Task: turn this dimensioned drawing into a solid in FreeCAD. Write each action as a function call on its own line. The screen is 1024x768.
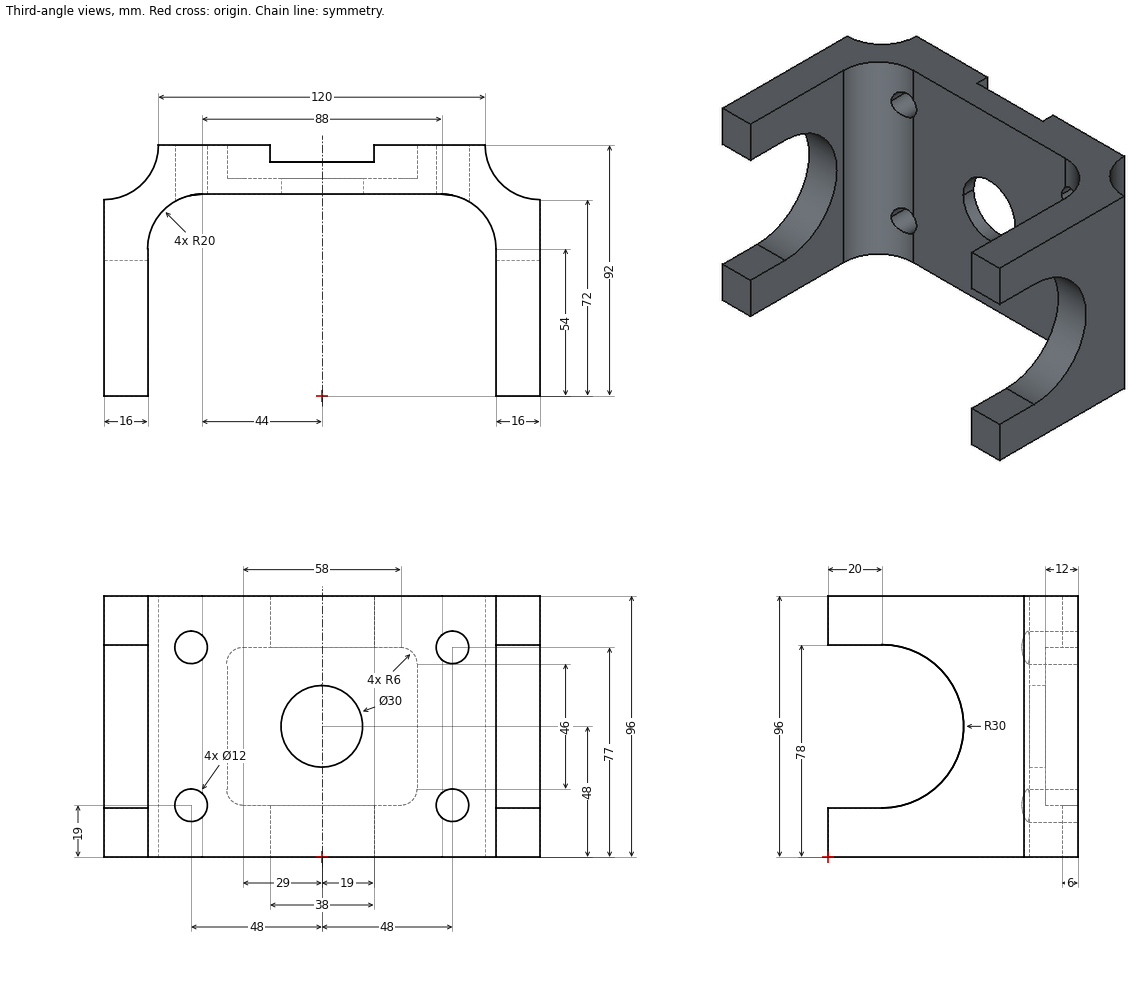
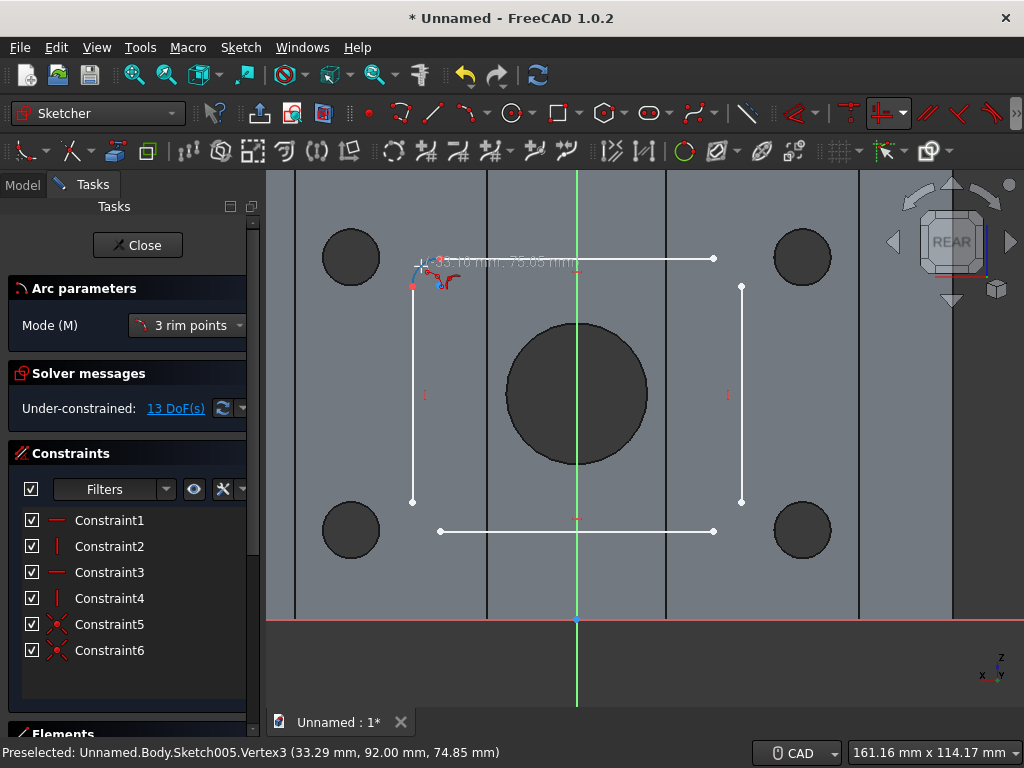
click(413, 503)
click(441, 532)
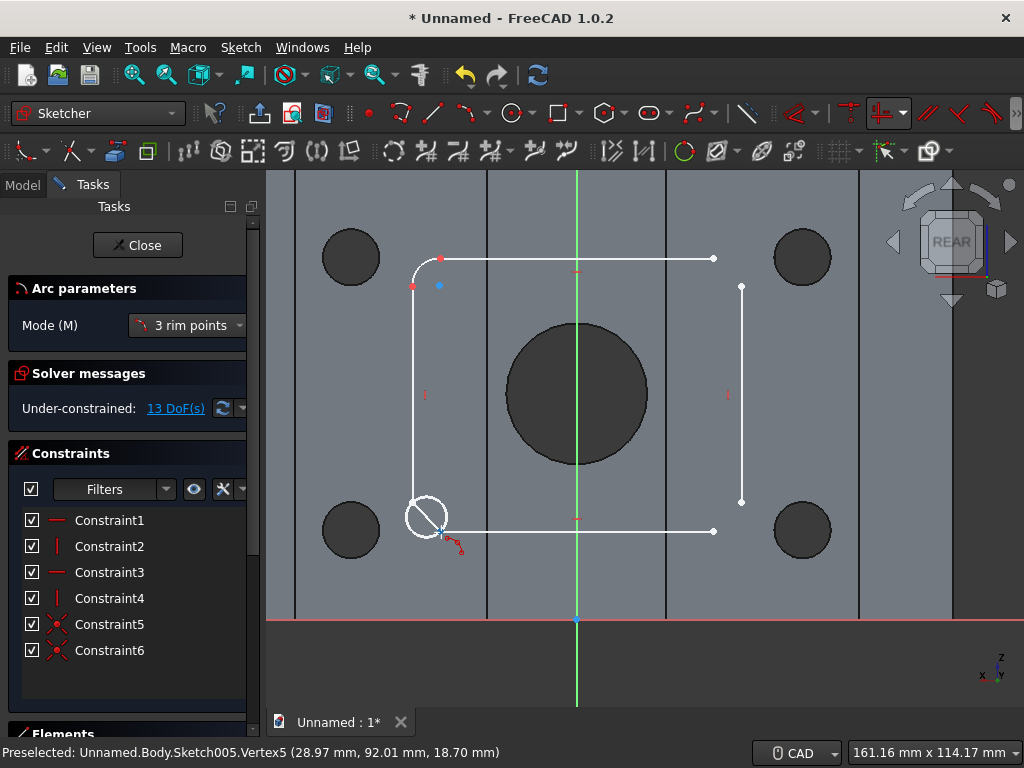
scroll(420, 522, up, 4)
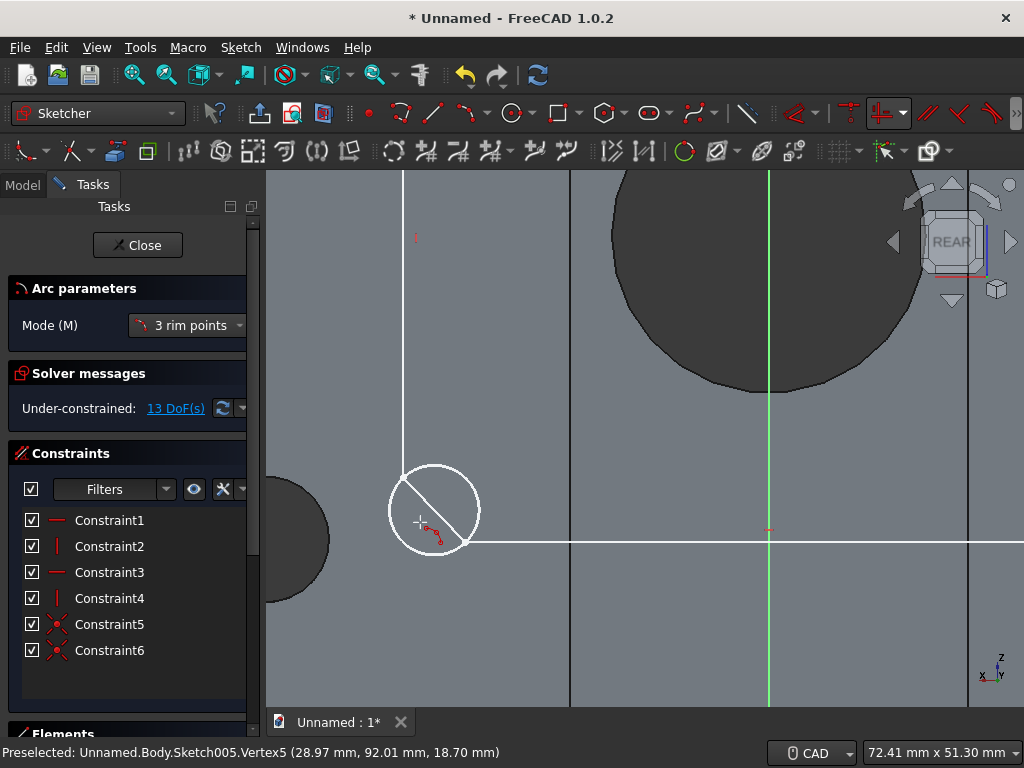
click(421, 521)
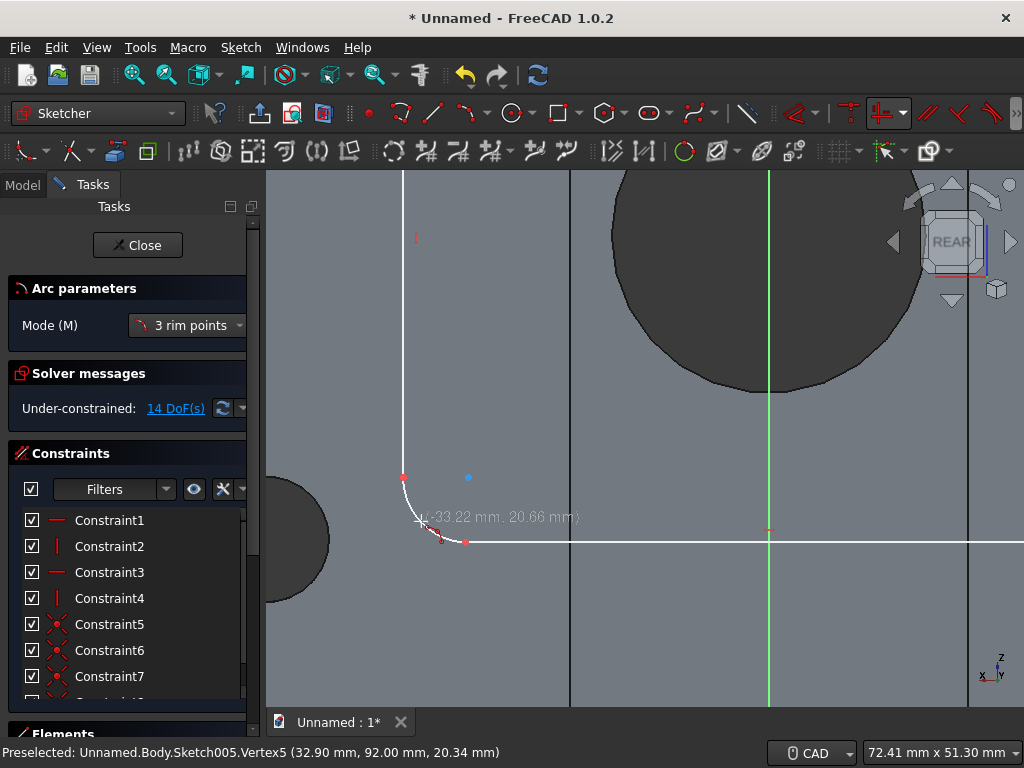
scroll(420, 523, down, 4)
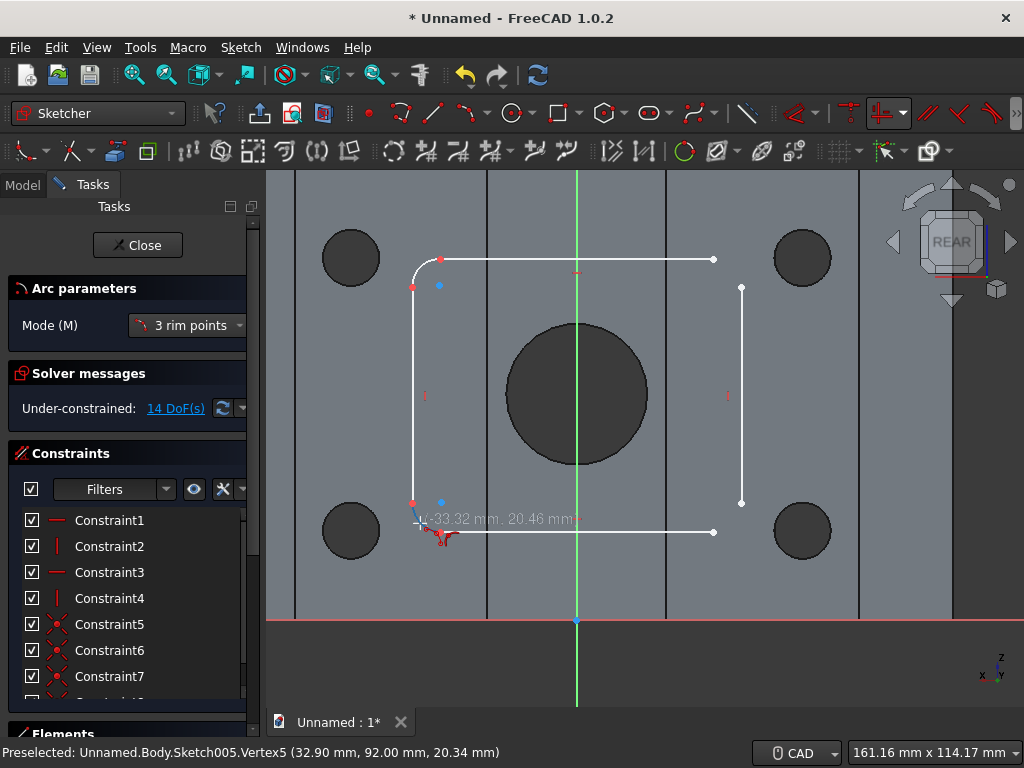
click(714, 532)
click(742, 503)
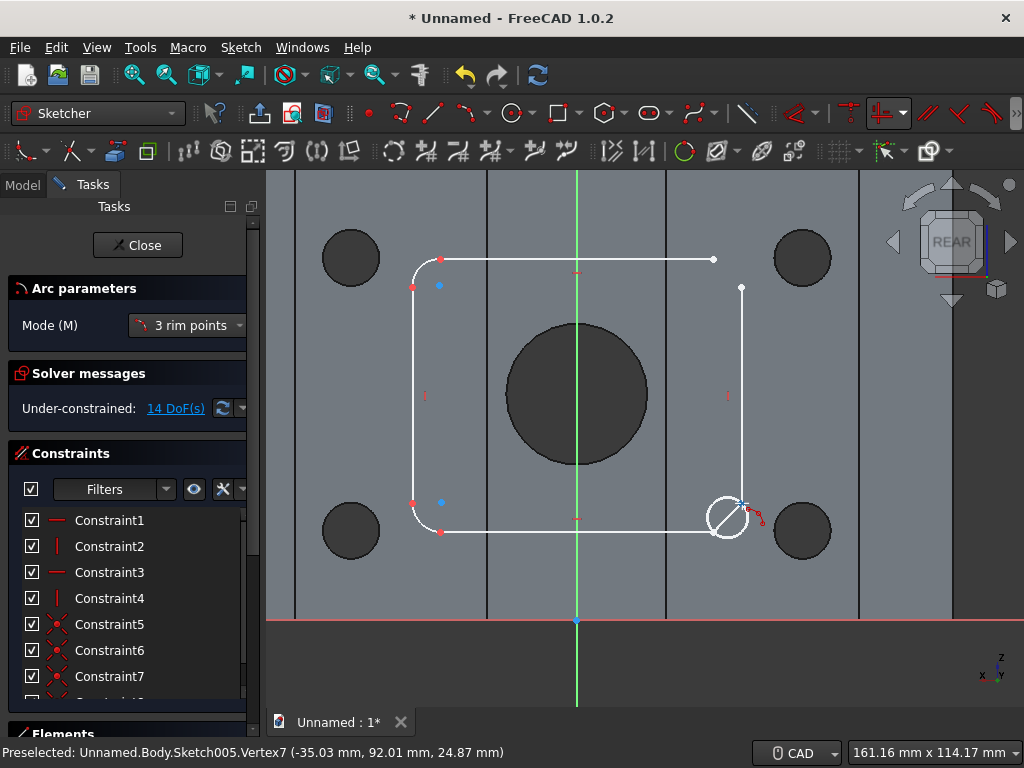
scroll(733, 522, up, 4)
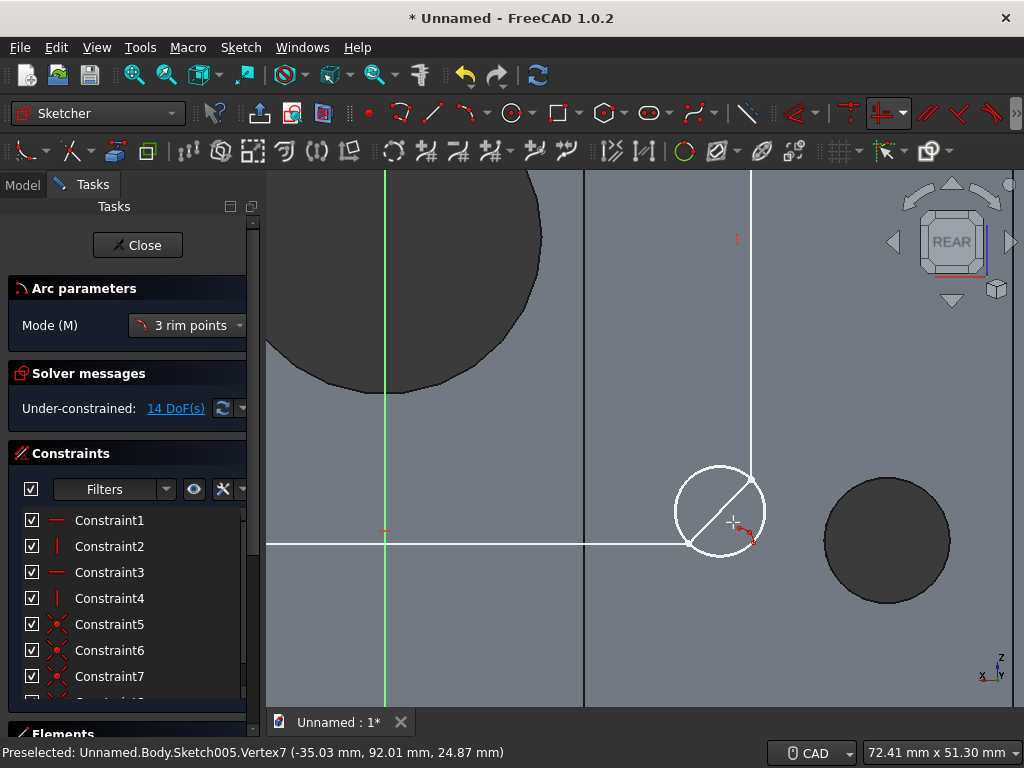
click(733, 522)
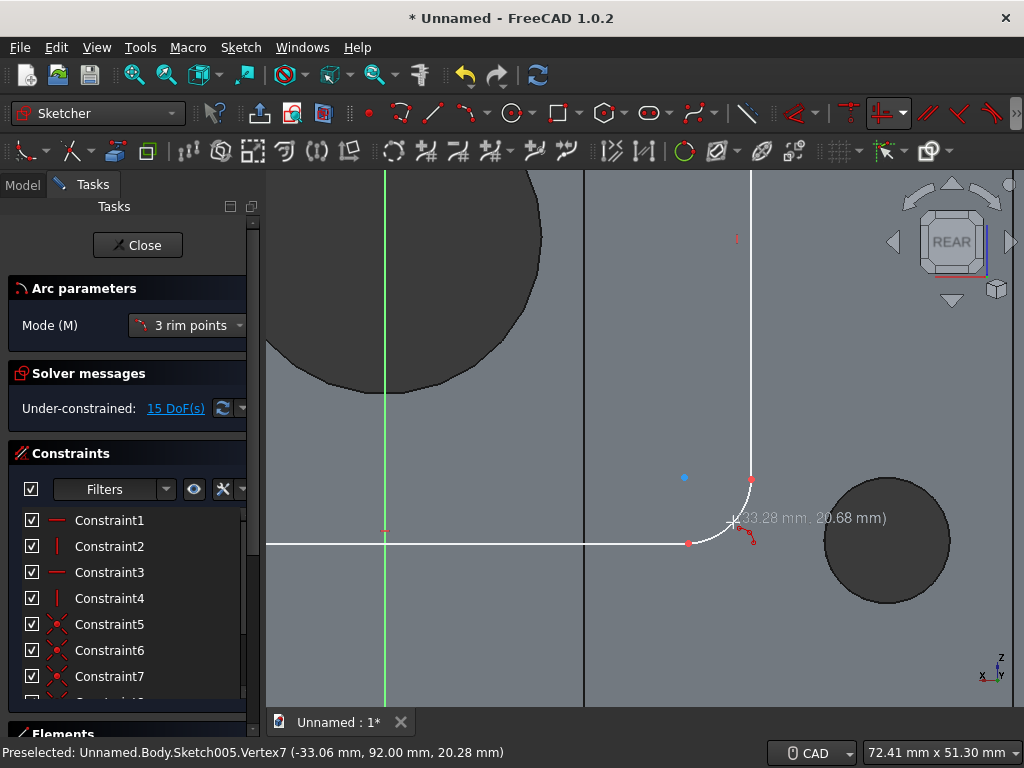
scroll(733, 522, down, 4)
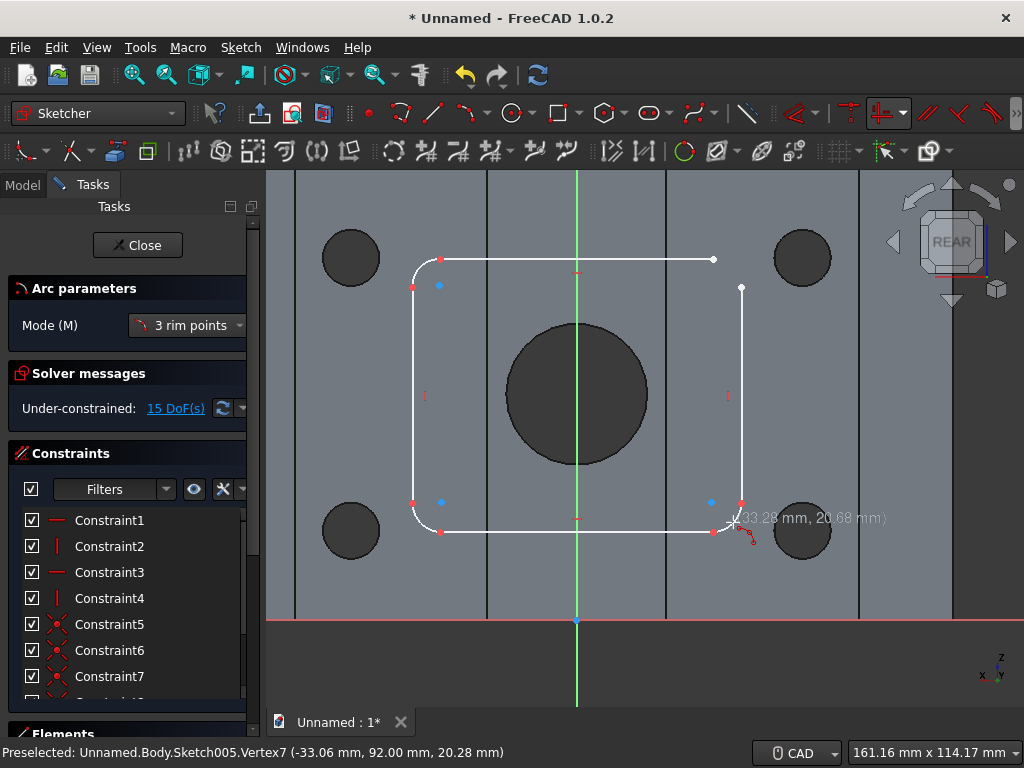
click(742, 287)
click(714, 259)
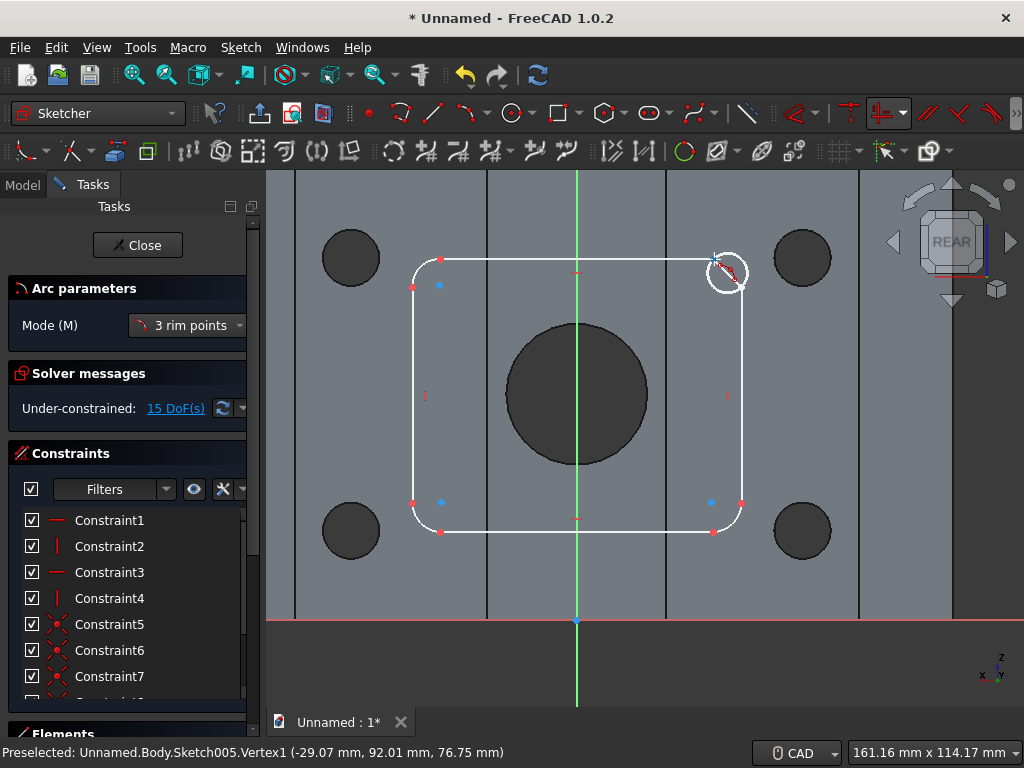
scroll(733, 266, up, 4)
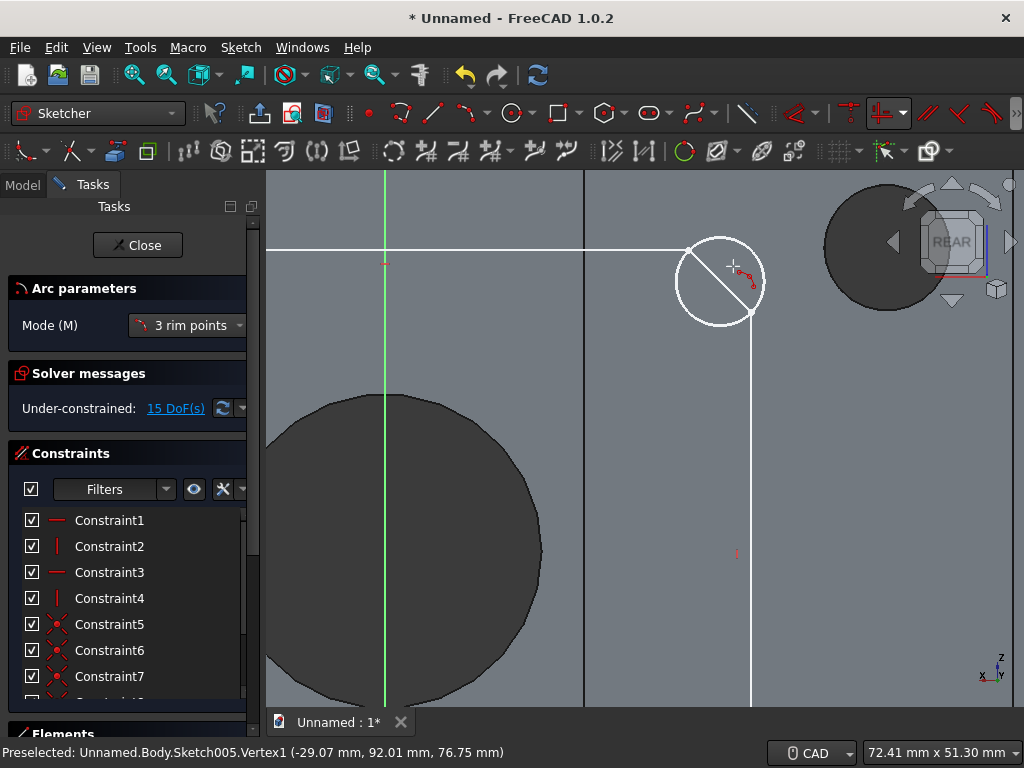
click(733, 266)
key(Escape)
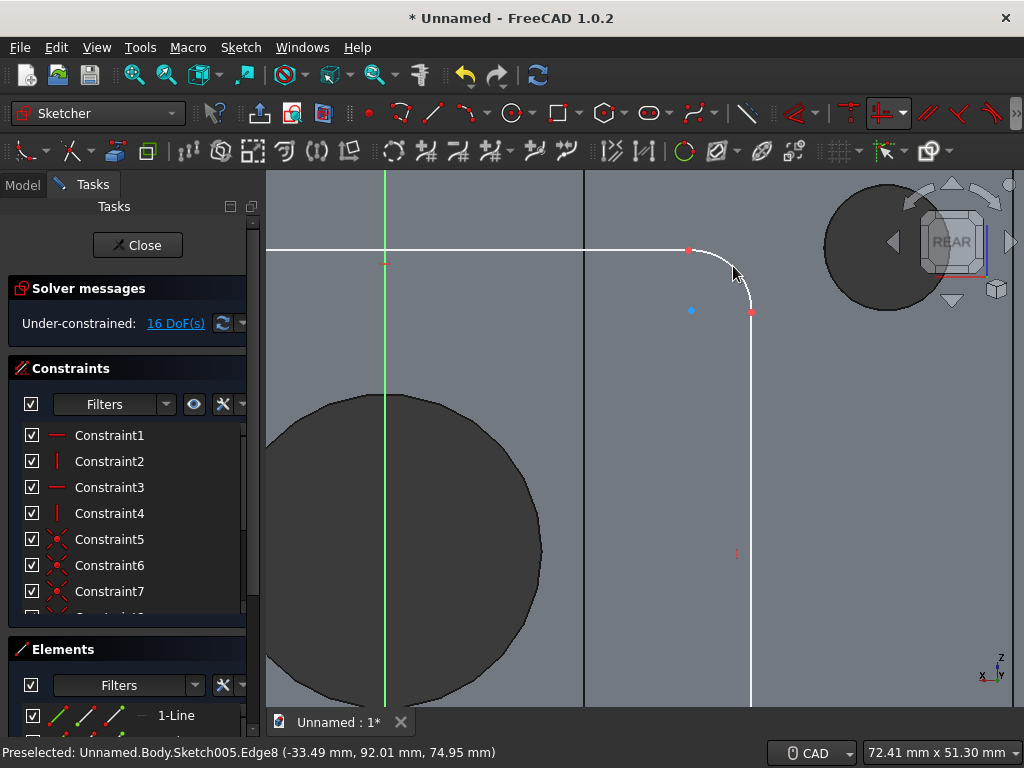
click(507, 250)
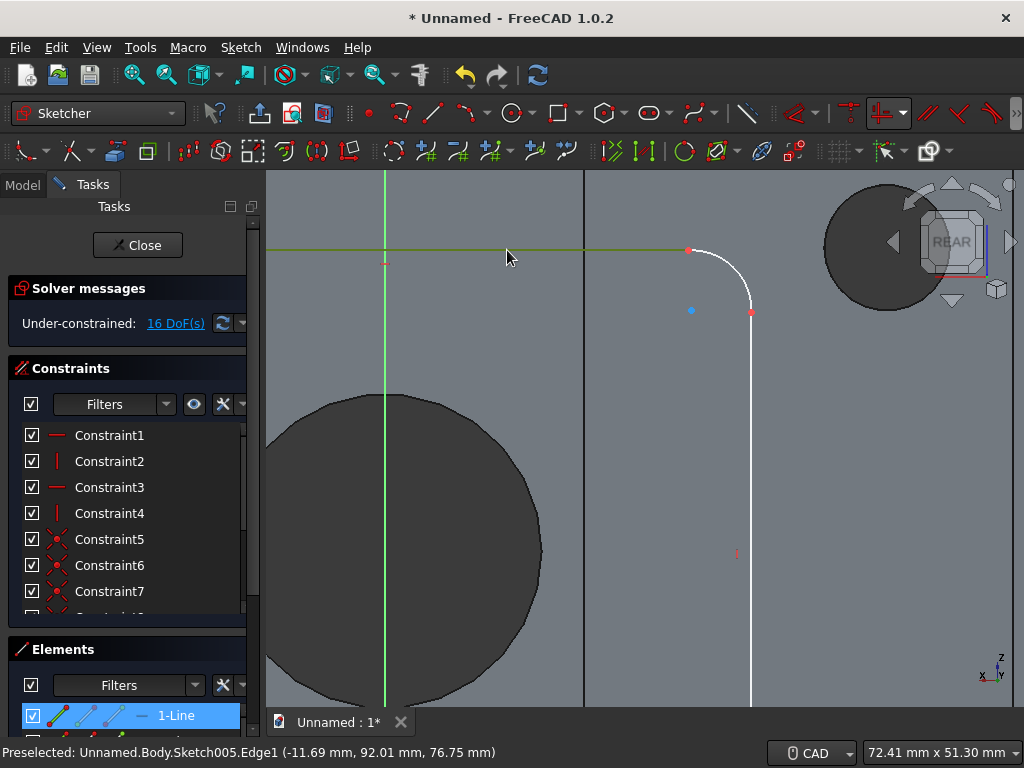
scroll(733, 265, down, 4)